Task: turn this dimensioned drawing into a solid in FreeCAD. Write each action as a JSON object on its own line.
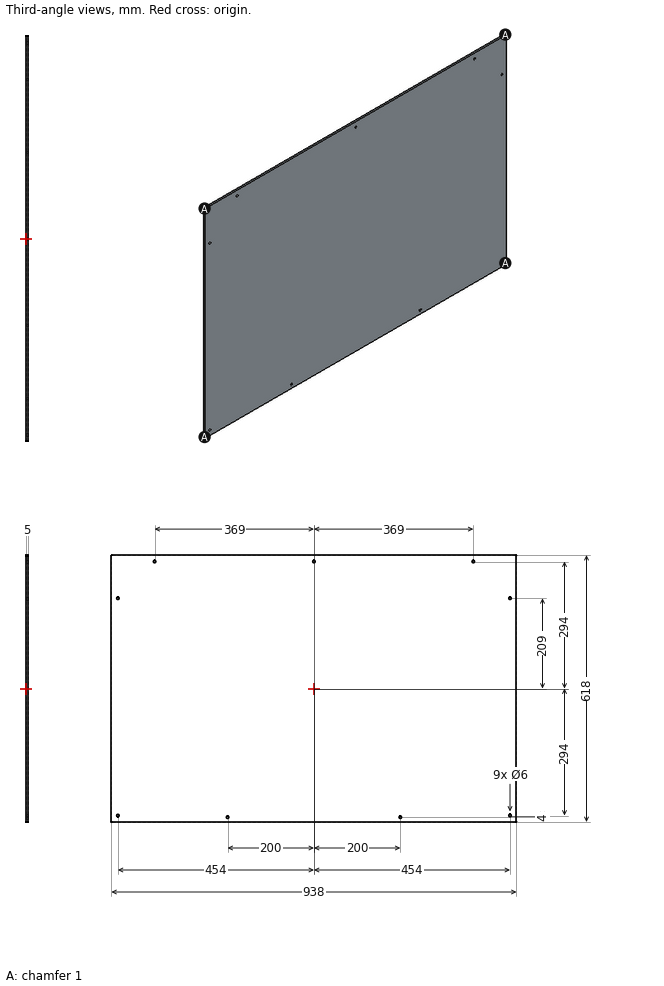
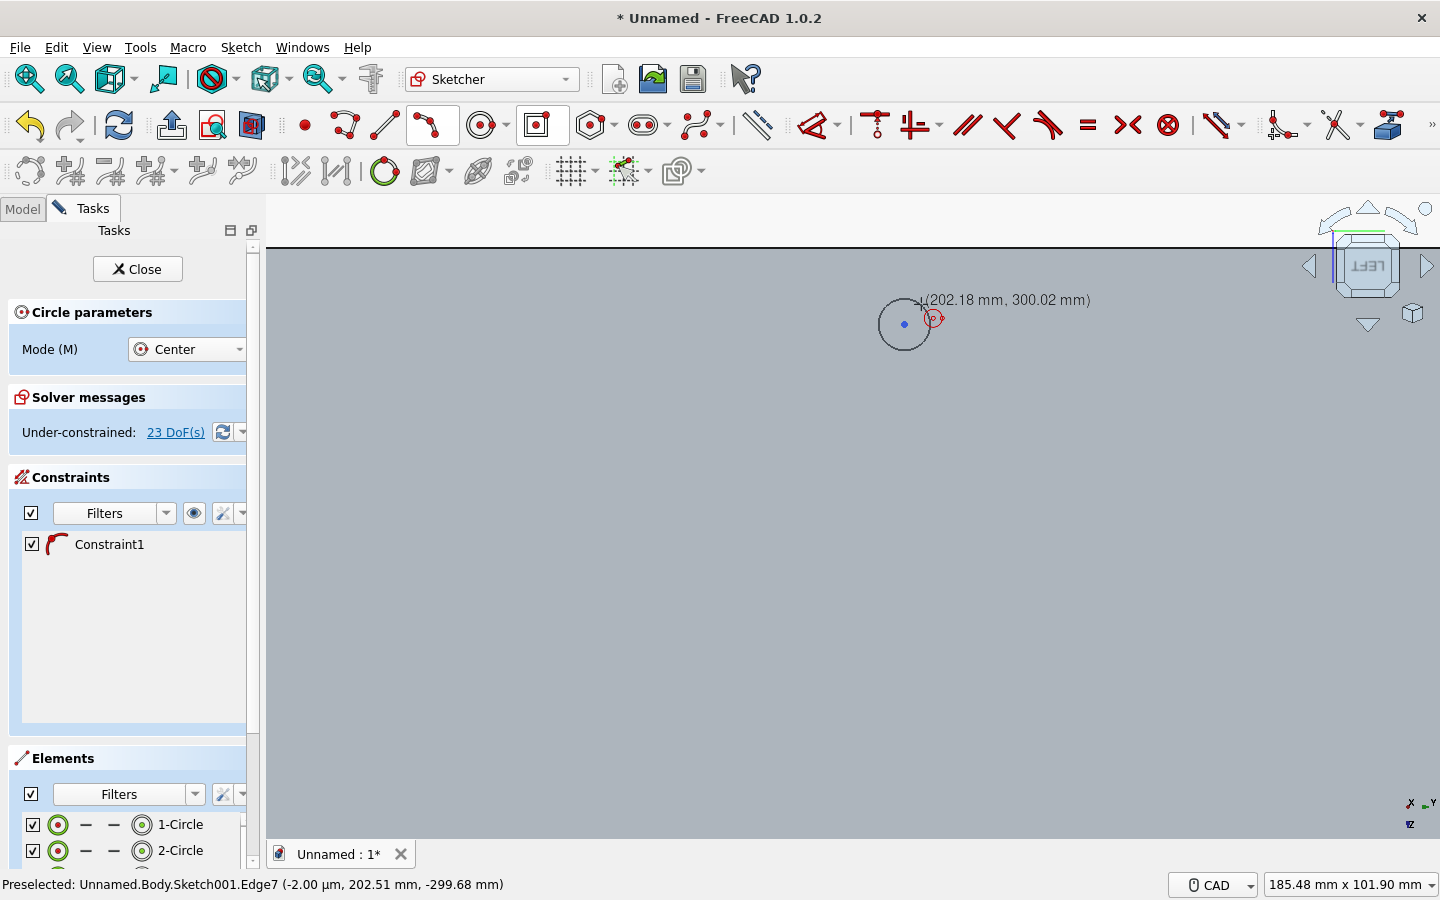
{"action": "scroll", "coordinate": [927, 308], "scroll_direction": "down", "scroll_amount": 11}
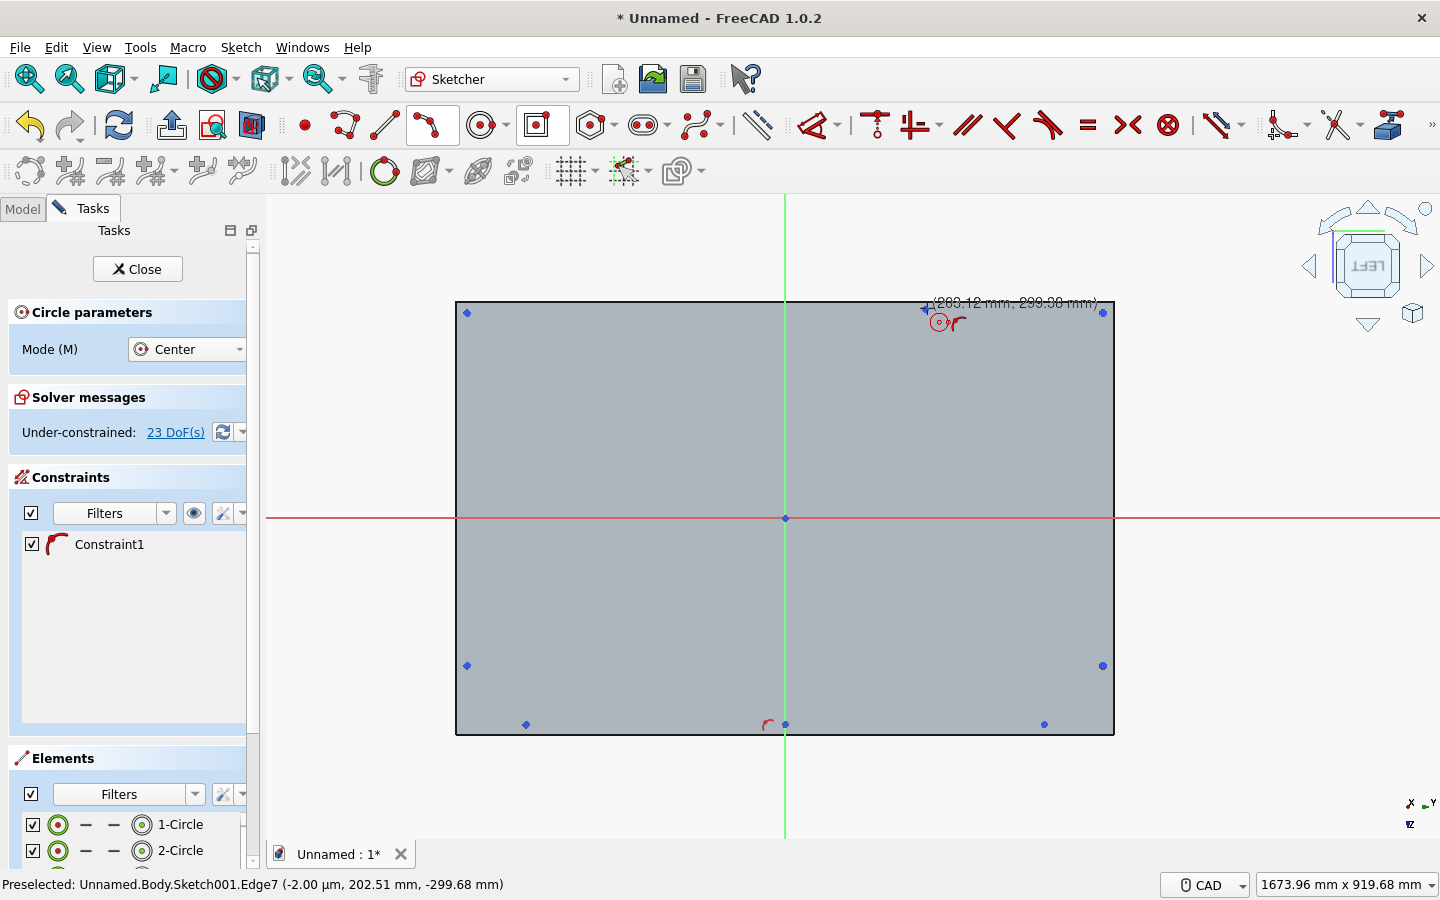
{"action": "scroll", "coordinate": [645, 309], "scroll_direction": "up", "scroll_amount": 12}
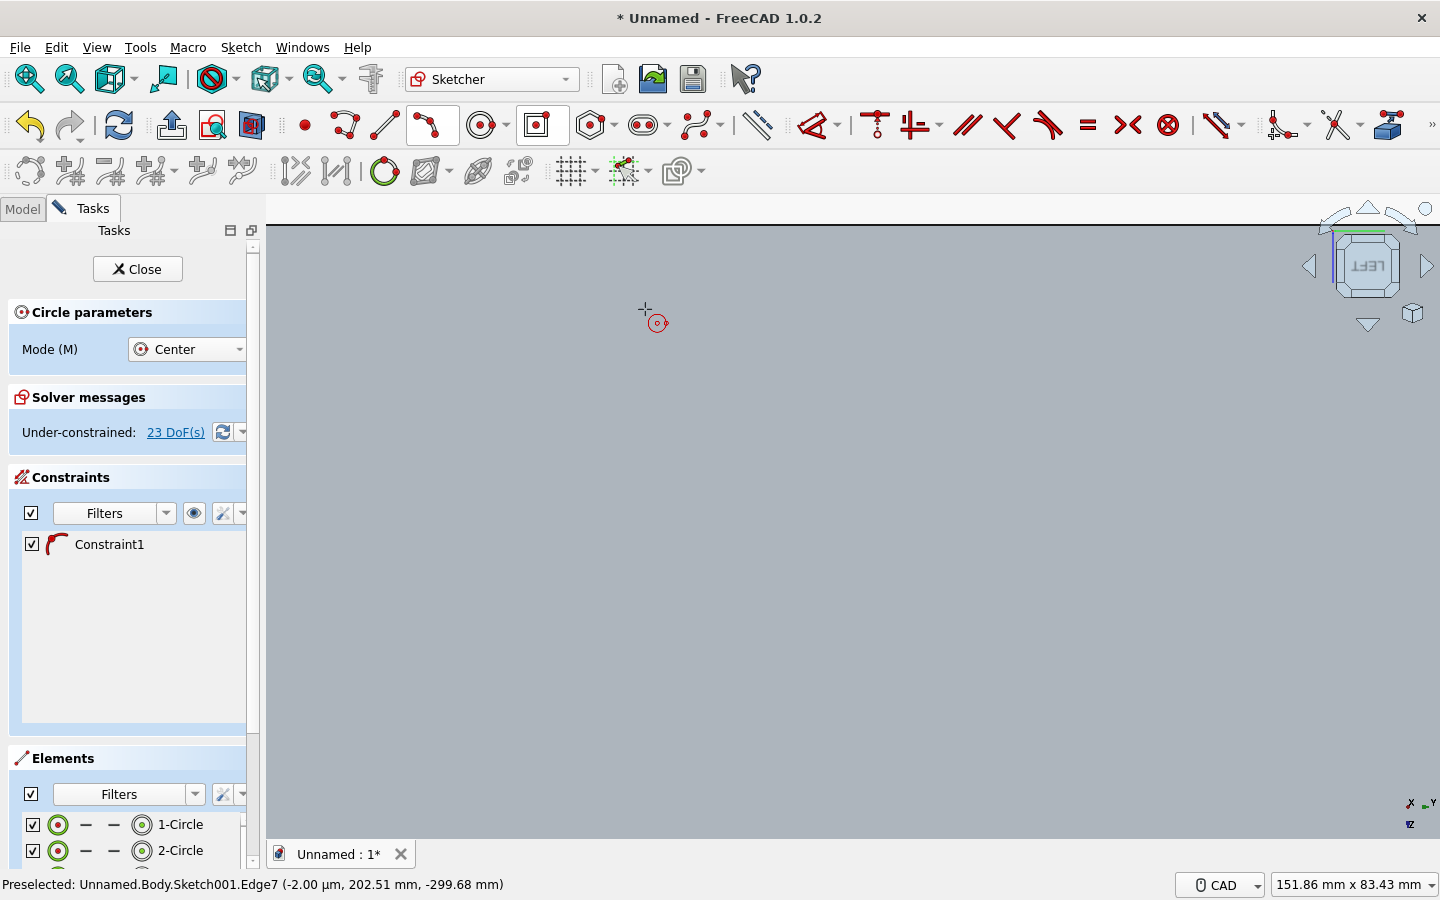
{"action": "scroll", "coordinate": [645, 309], "scroll_direction": "down", "scroll_amount": 12}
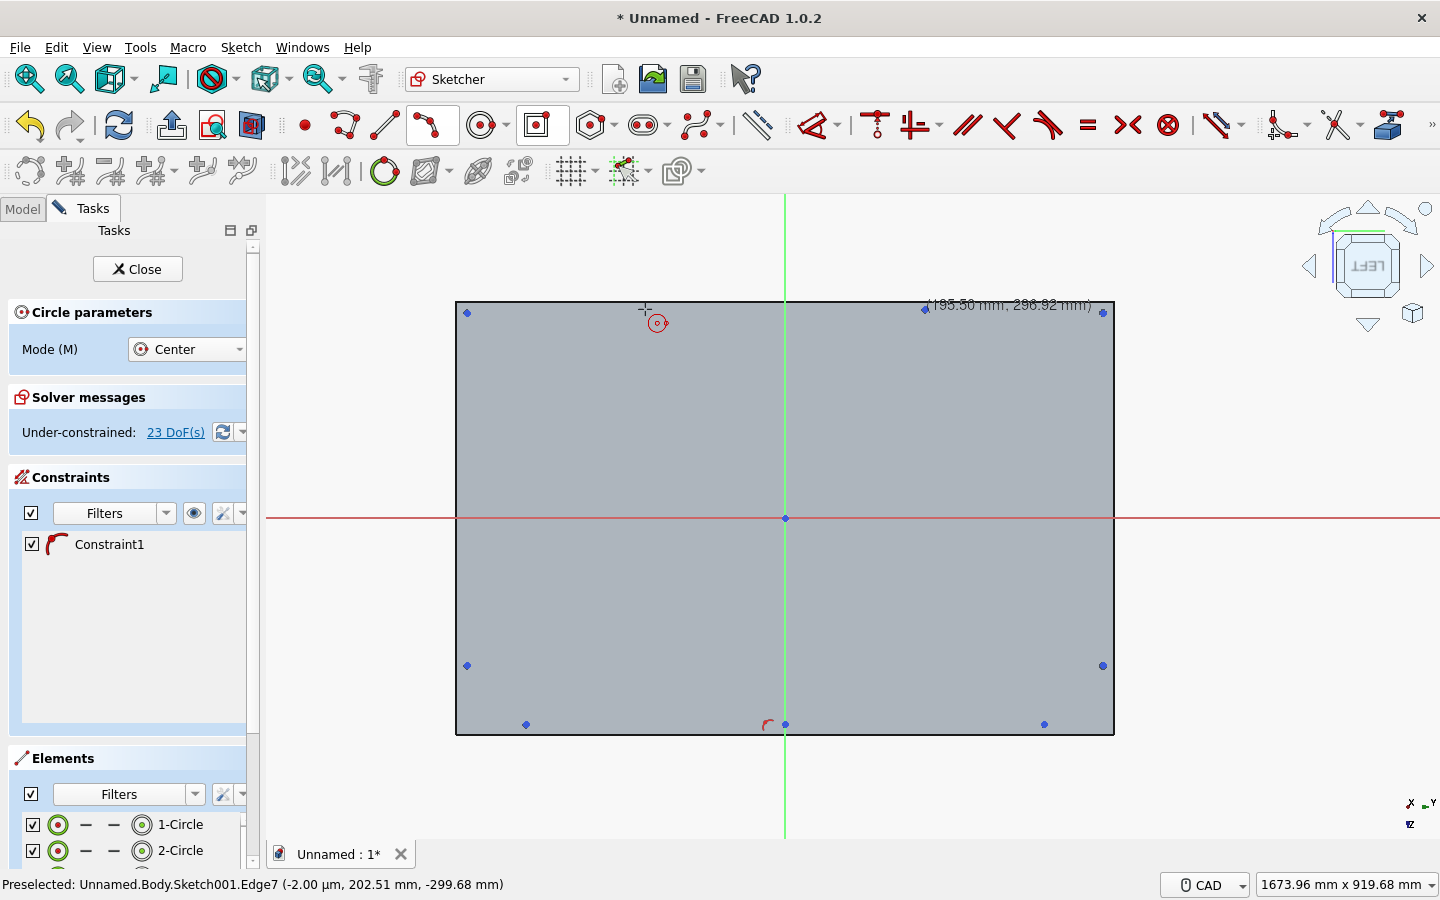
{"action": "left_click", "coordinate": [645, 309]}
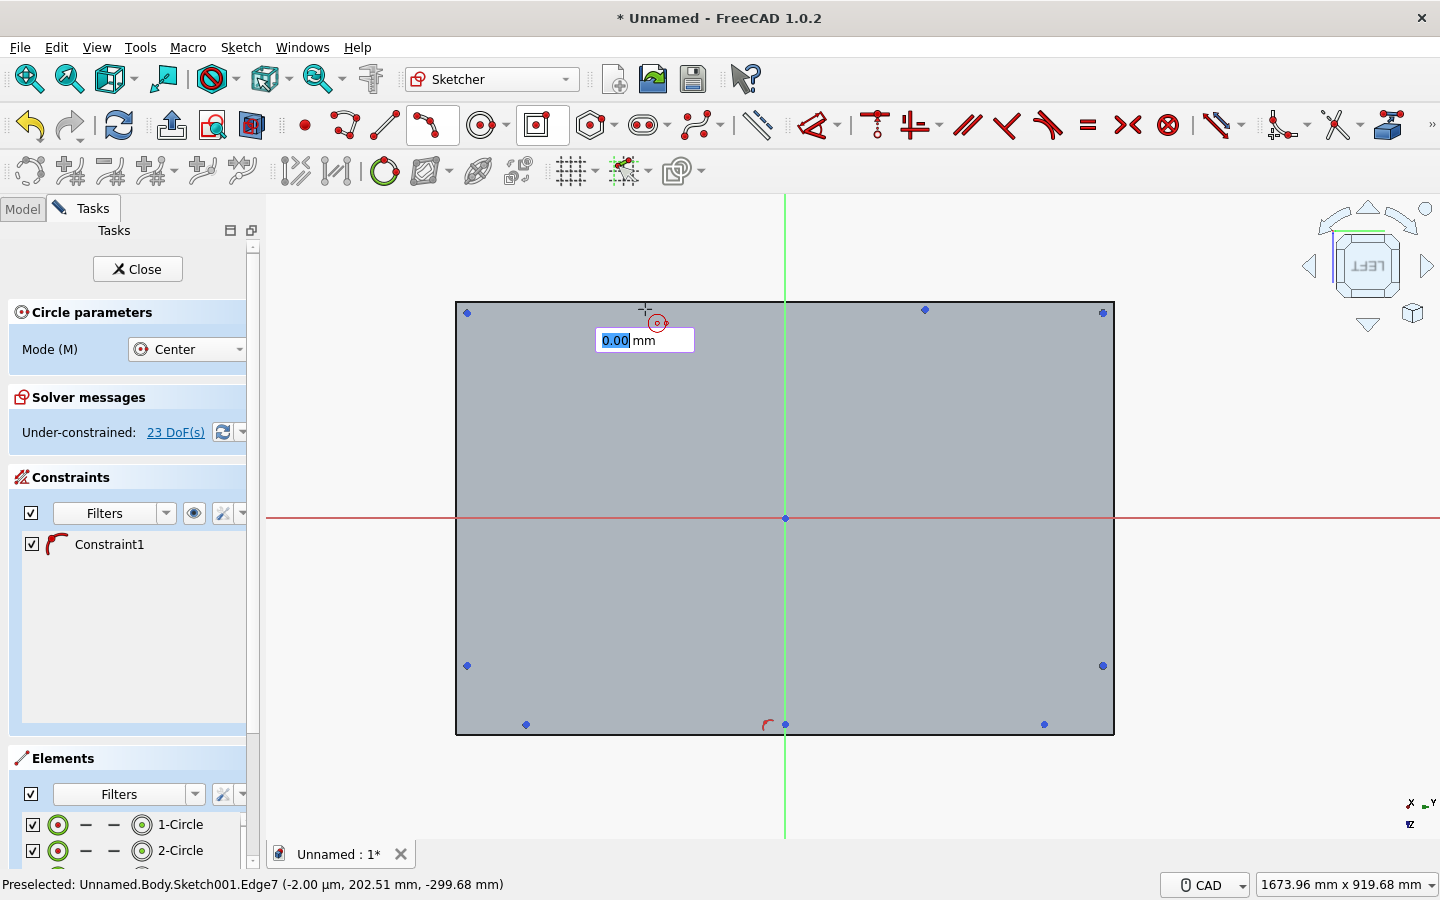
{"action": "scroll", "coordinate": [646, 308], "scroll_direction": "up", "scroll_amount": 11}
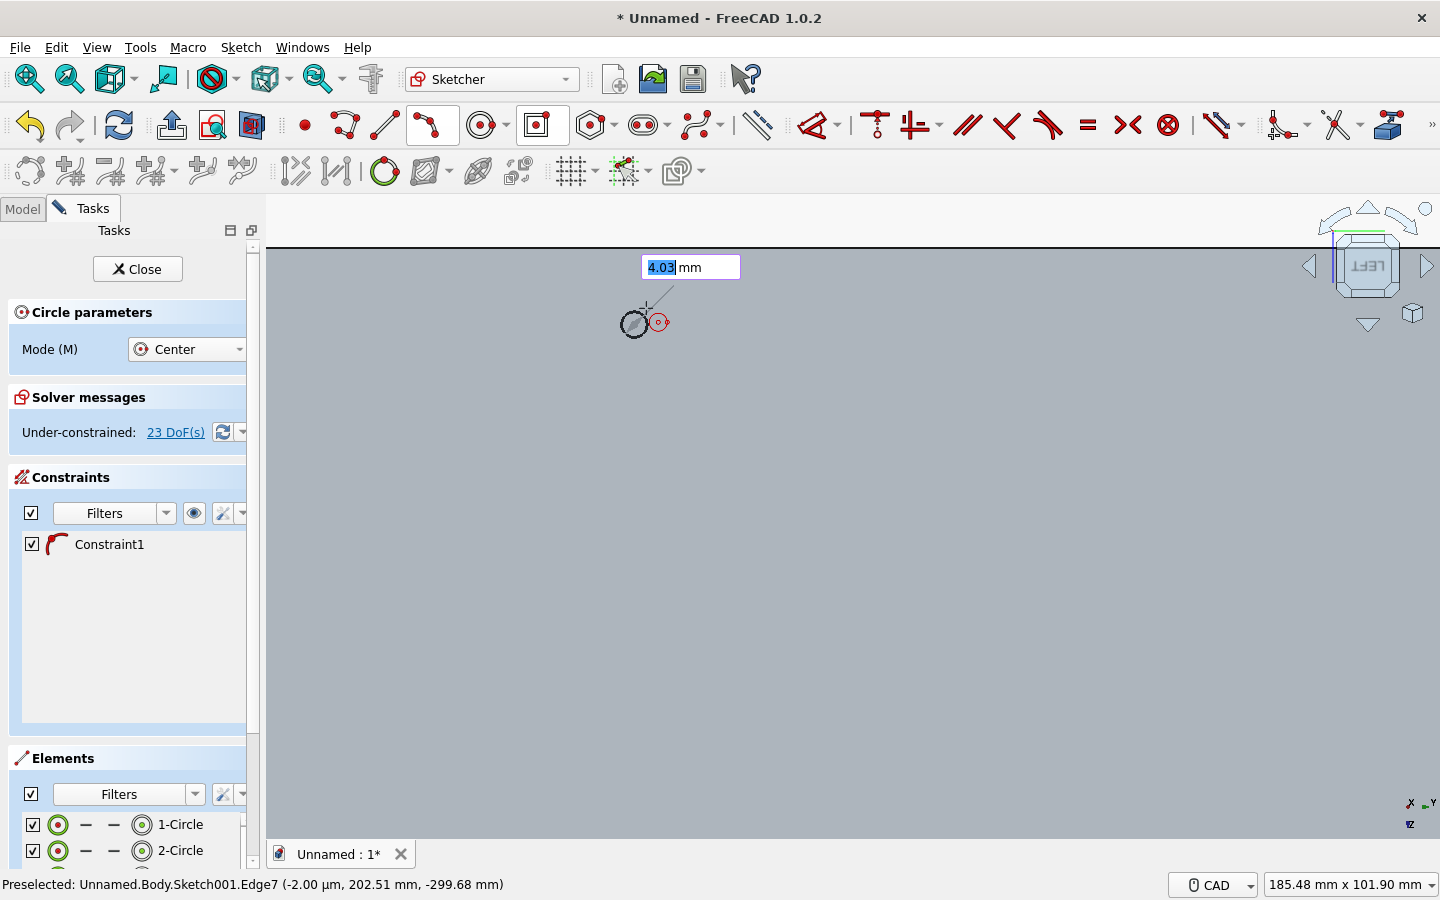
{"action": "left_click", "coordinate": [646, 304]}
{"action": "key", "text": "Escape"}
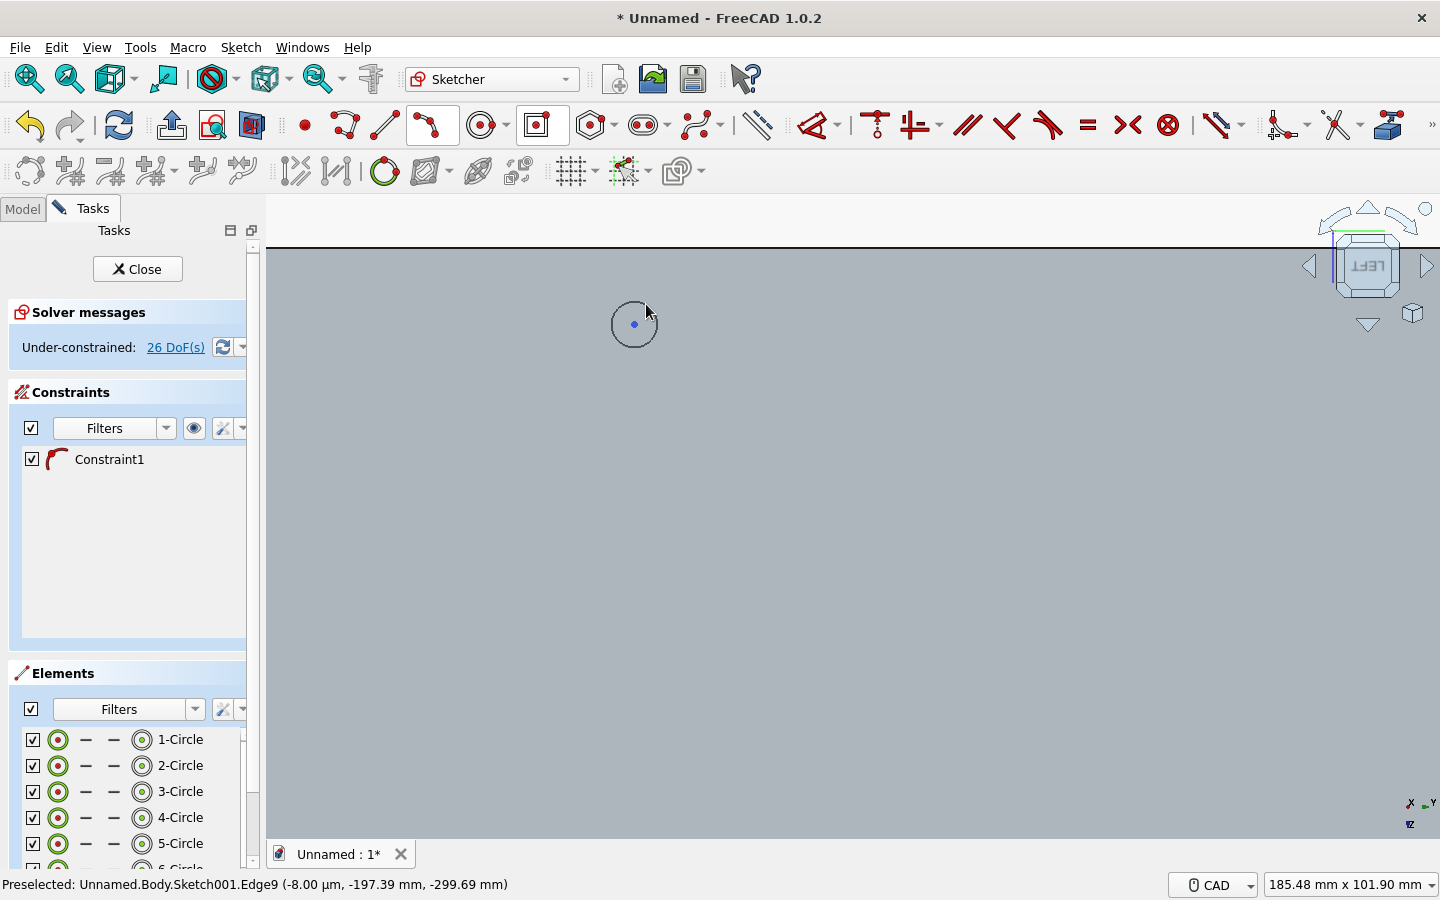
{"action": "scroll", "coordinate": [646, 308], "scroll_direction": "down", "scroll_amount": 11}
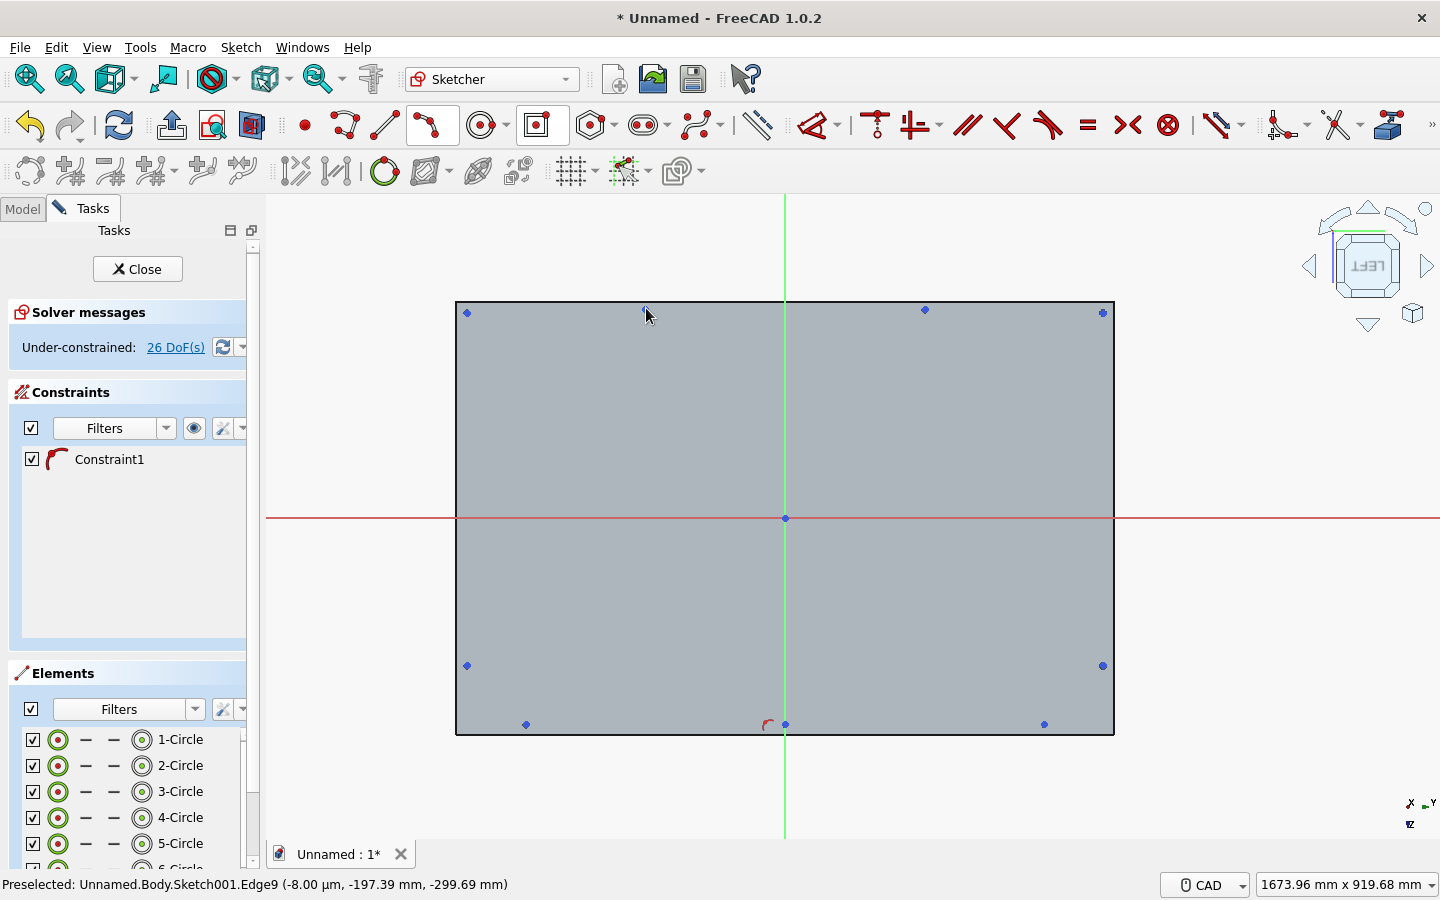
{"action": "scroll", "coordinate": [1105, 311], "scroll_direction": "up", "scroll_amount": 8}